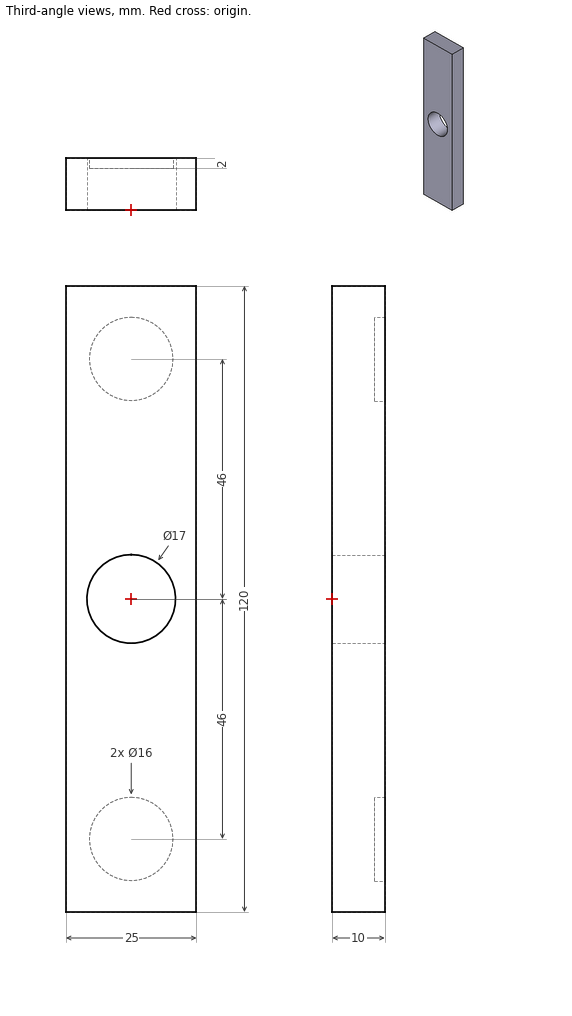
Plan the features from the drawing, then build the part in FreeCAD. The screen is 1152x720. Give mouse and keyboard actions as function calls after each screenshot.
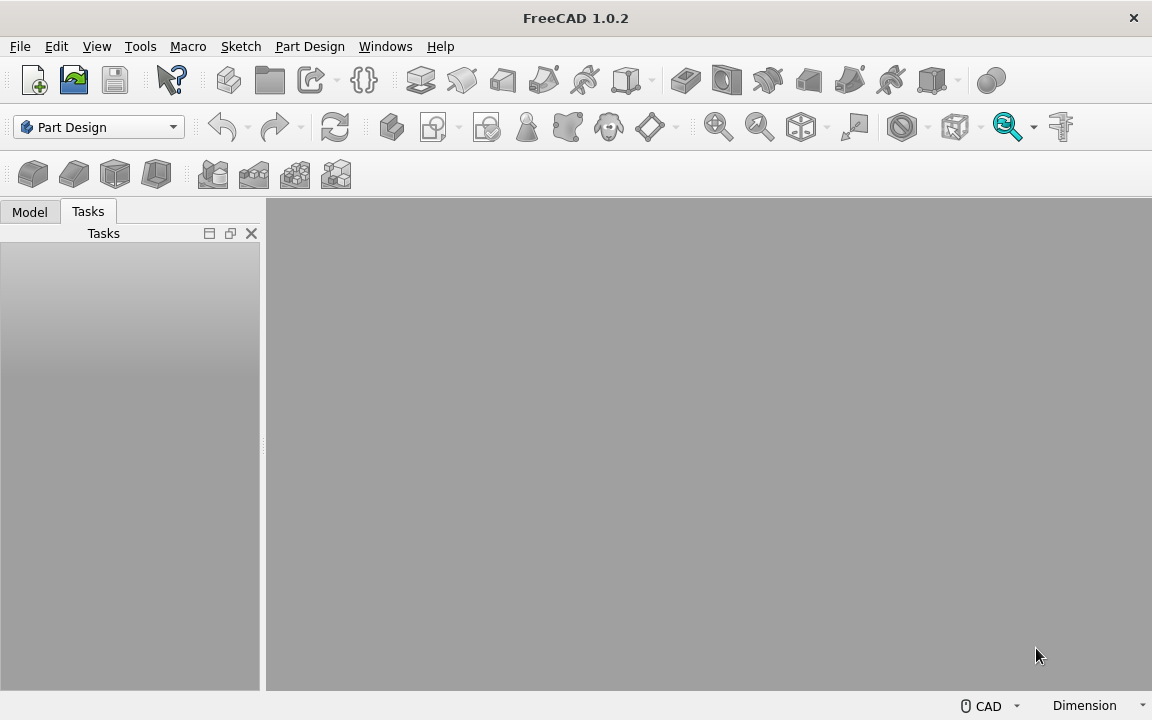
click(33, 80)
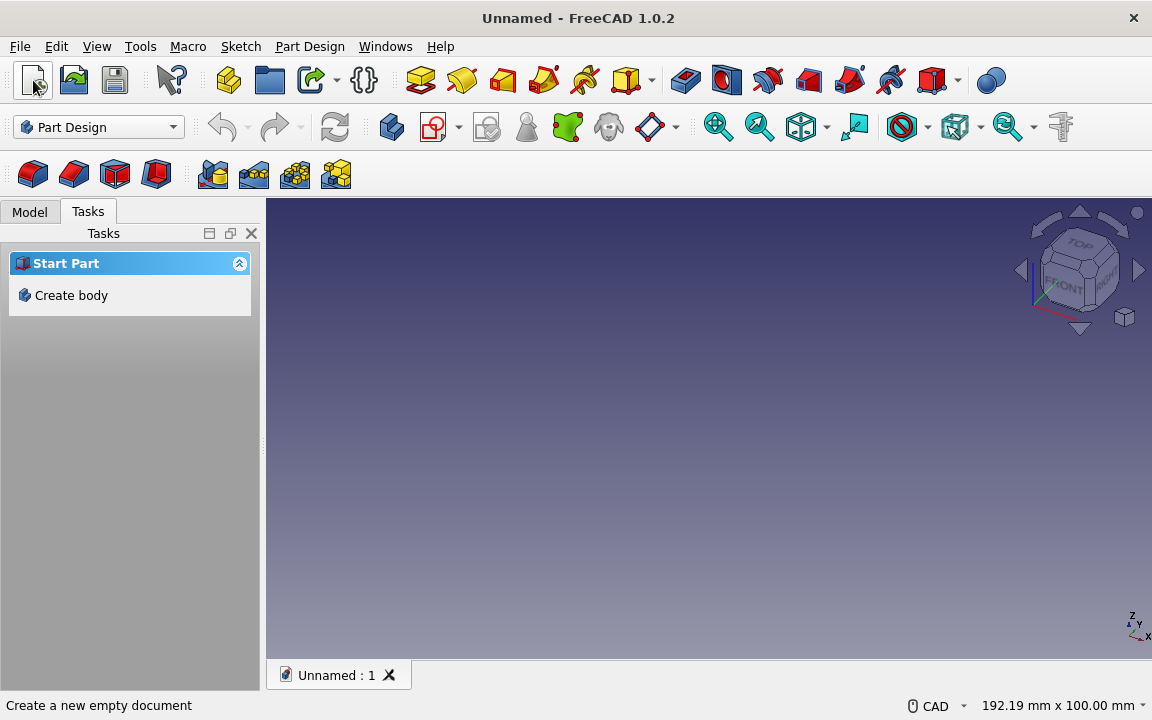
click(432, 128)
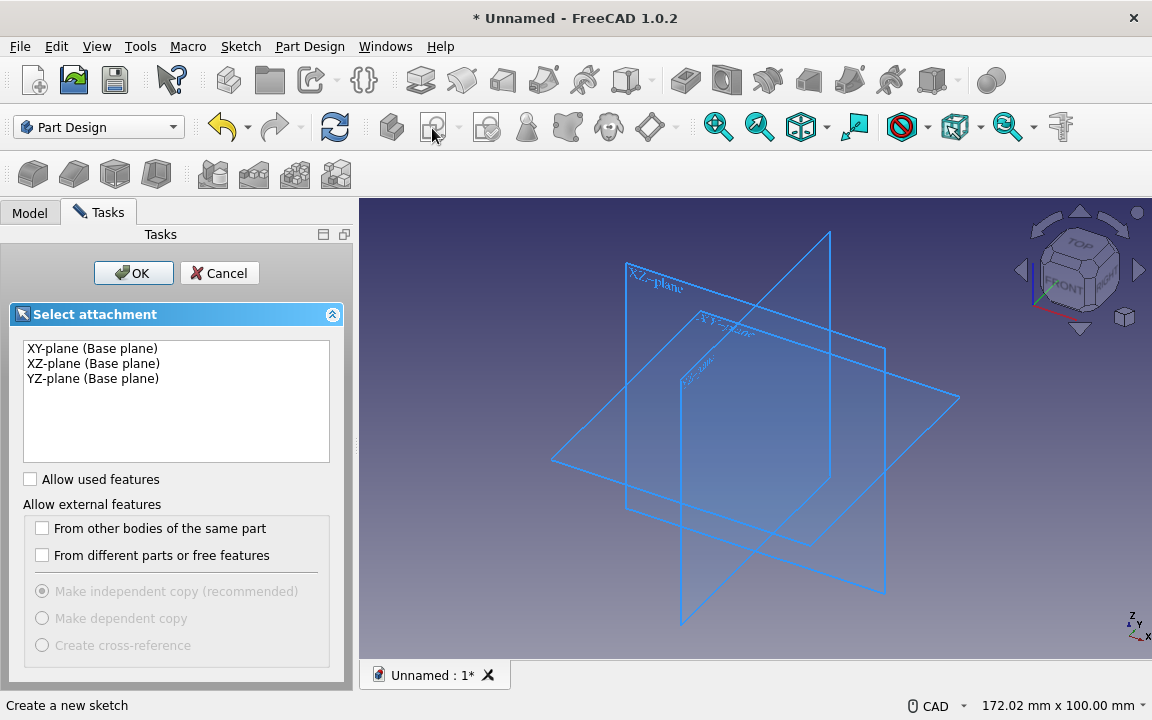
click(84, 364)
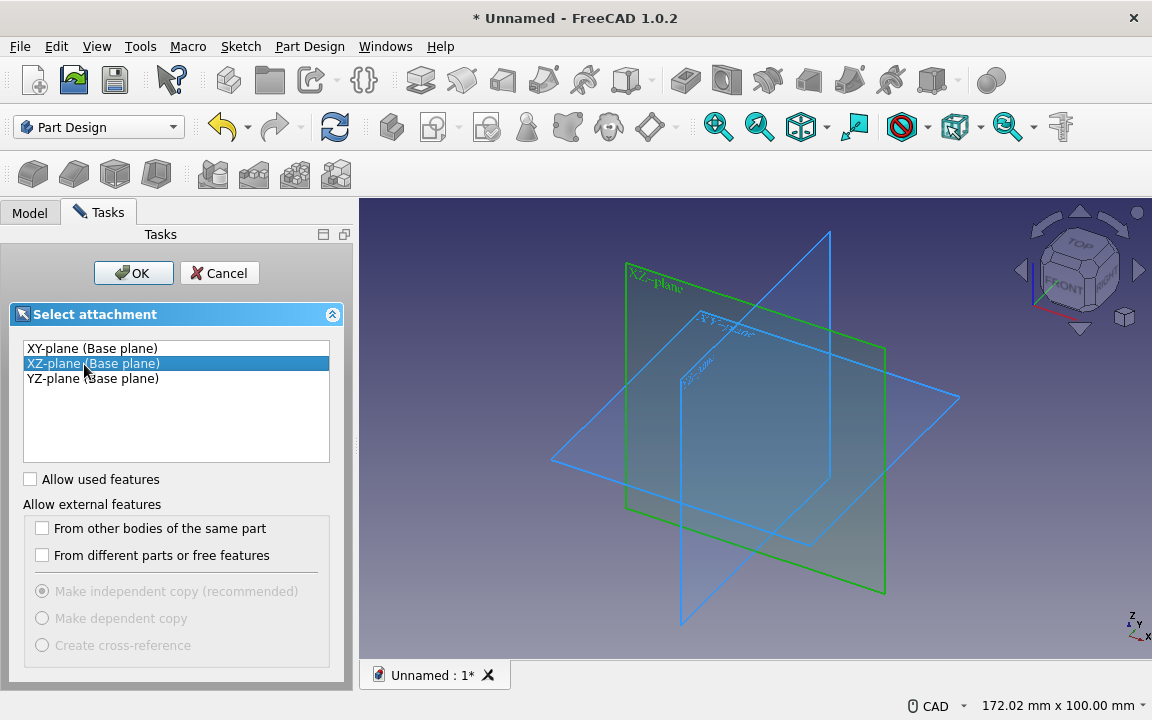
click(134, 273)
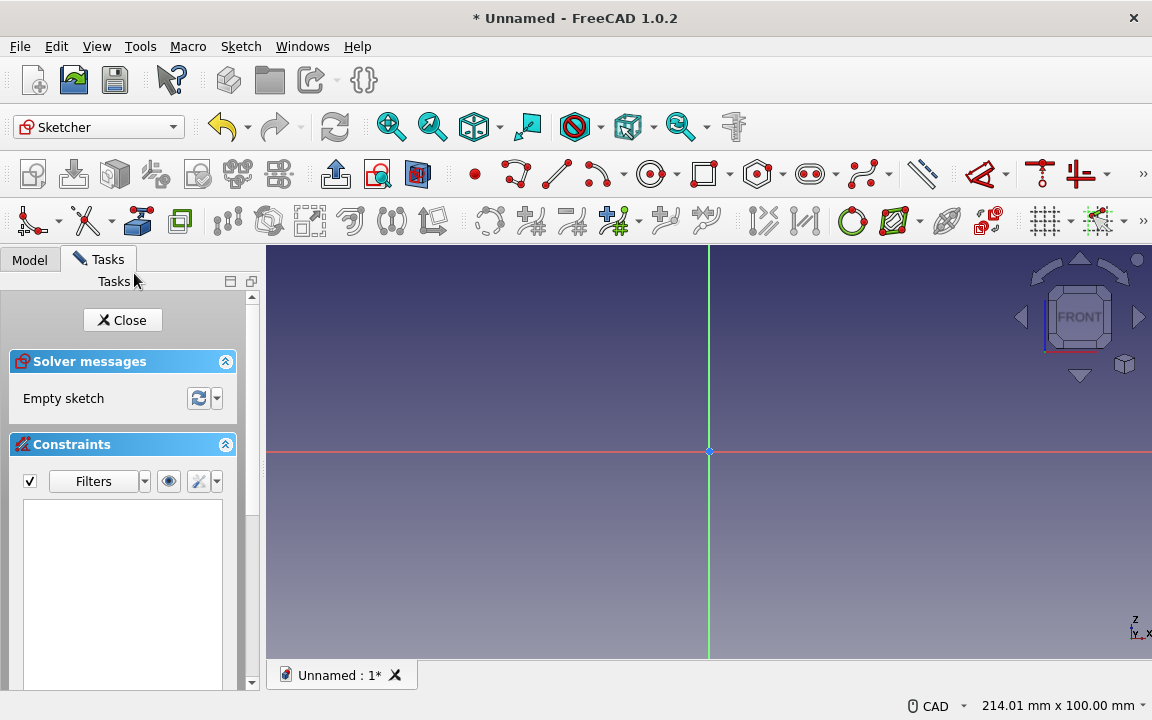
scroll(557, 452, down, 3)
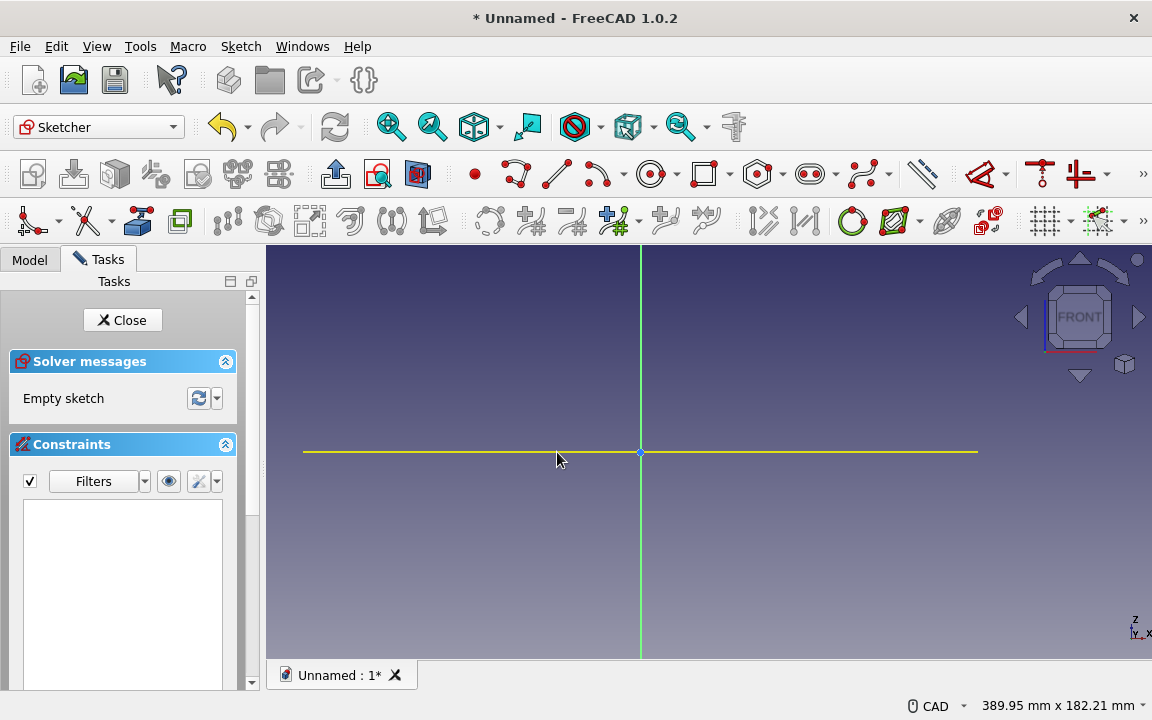
key(g)
key(v)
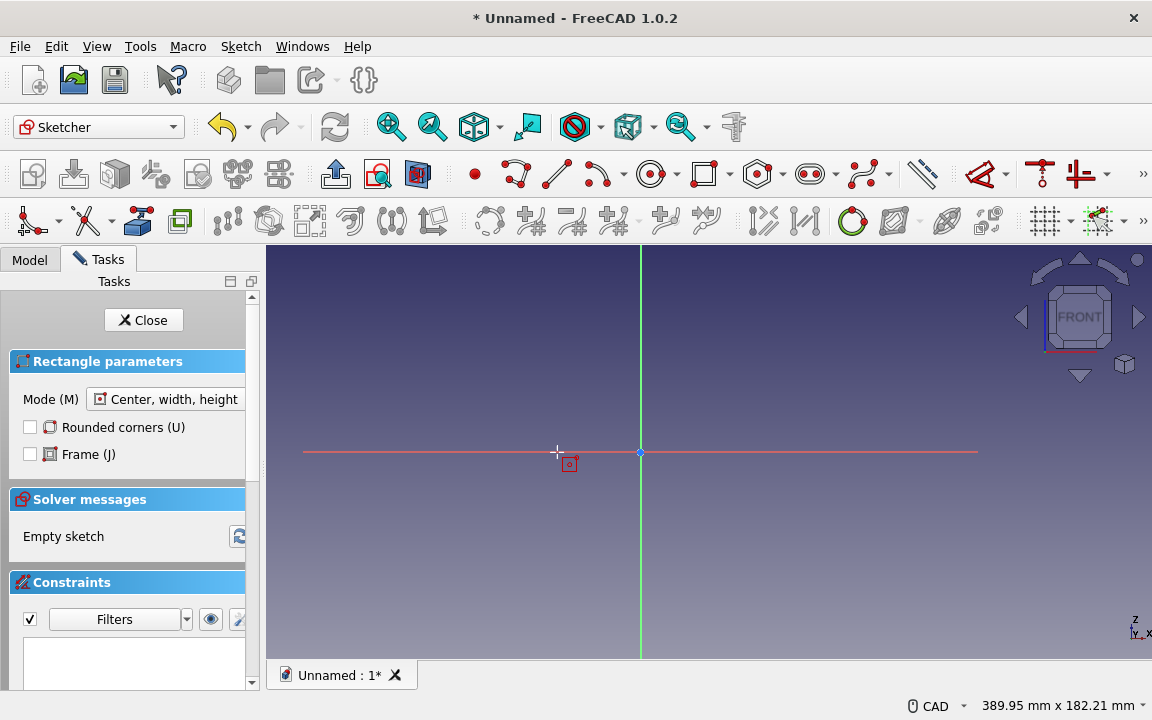
click(641, 452)
move(669, 316)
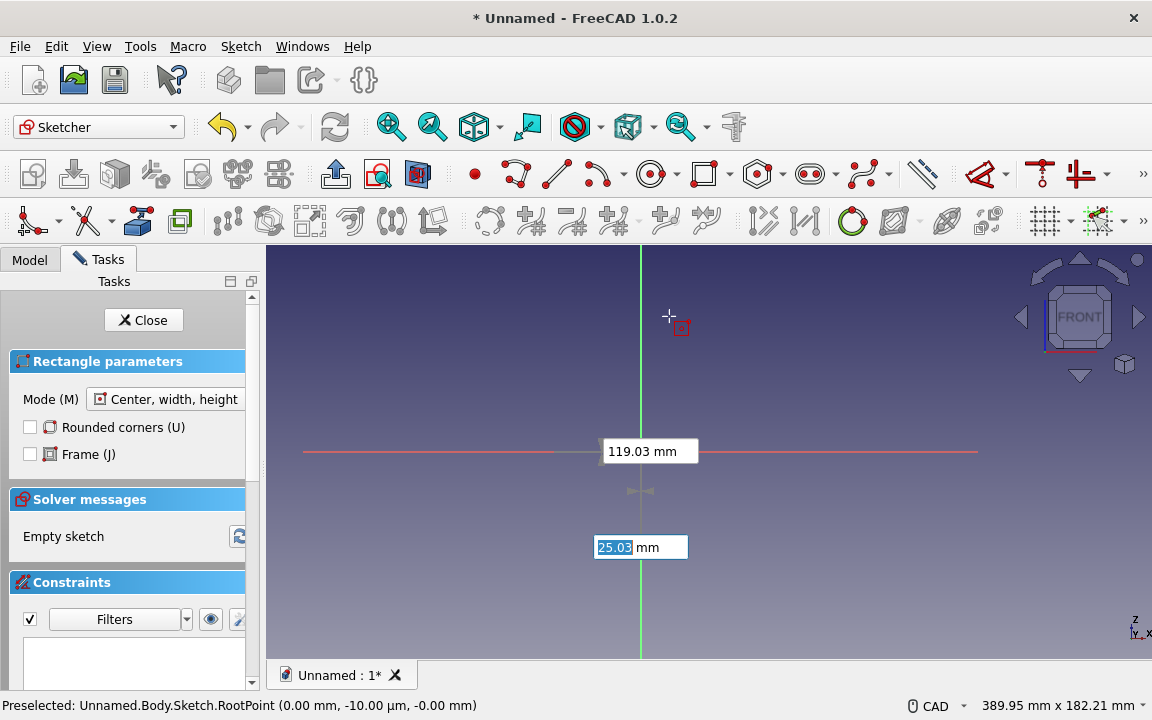
text(25)
key(Tab)
text(120)
key(Return)
key(Escape)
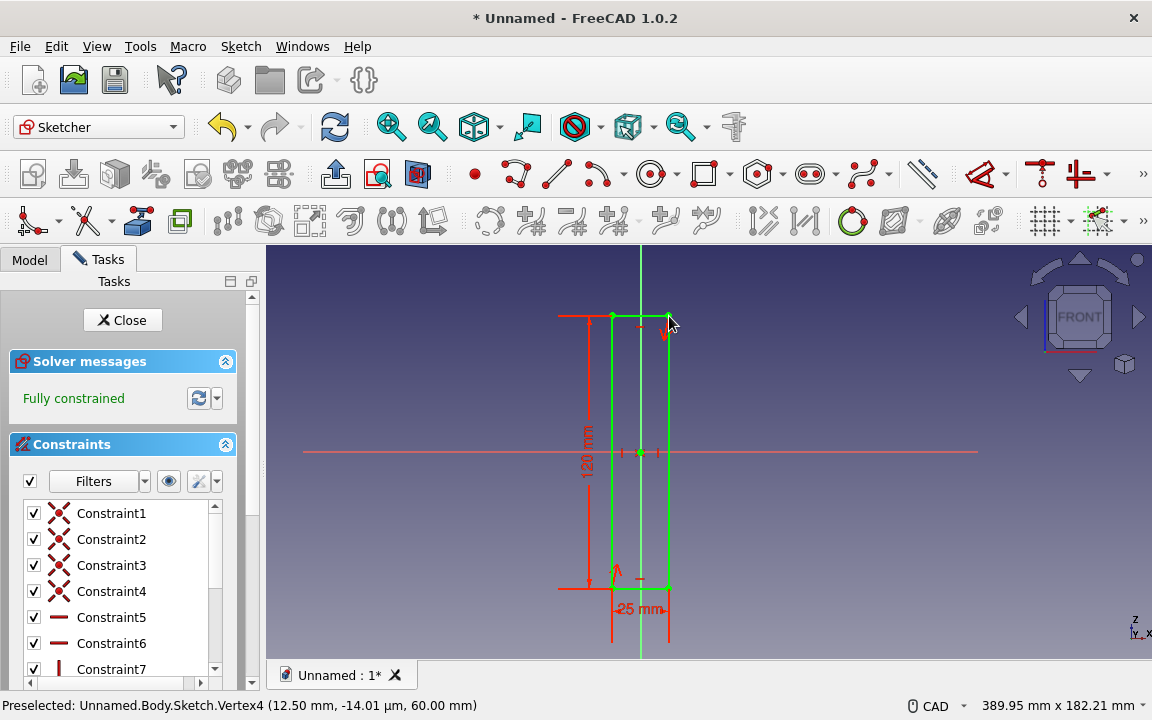
click(123, 320)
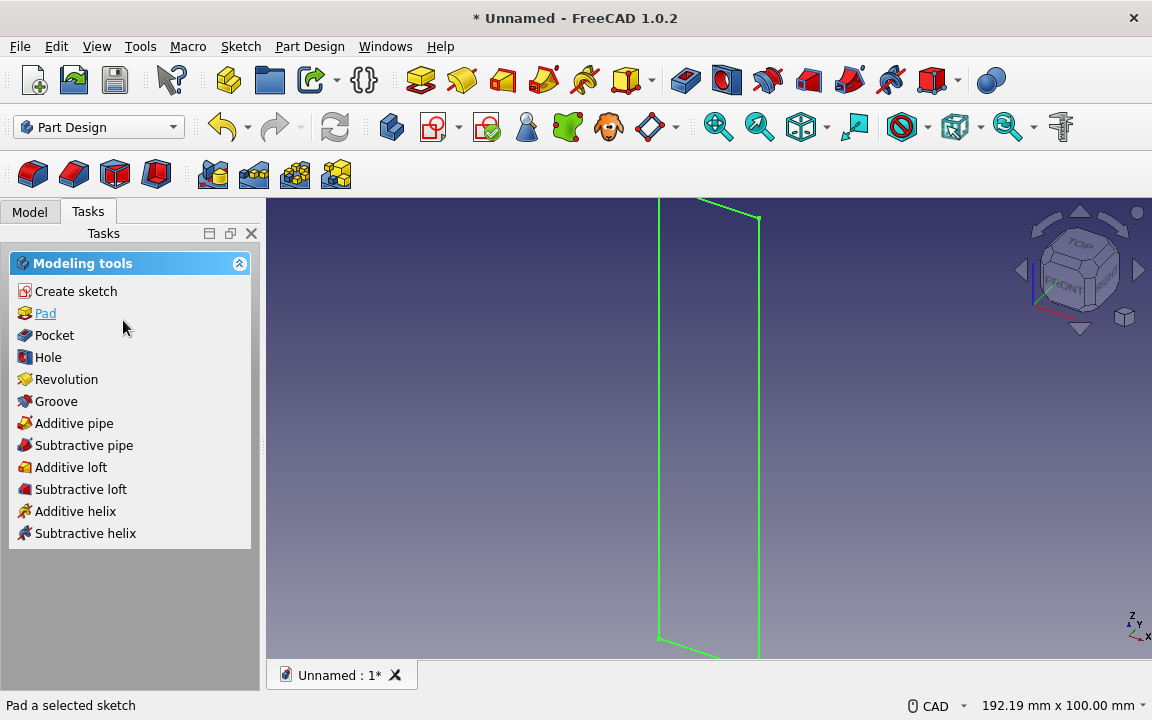
click(421, 80)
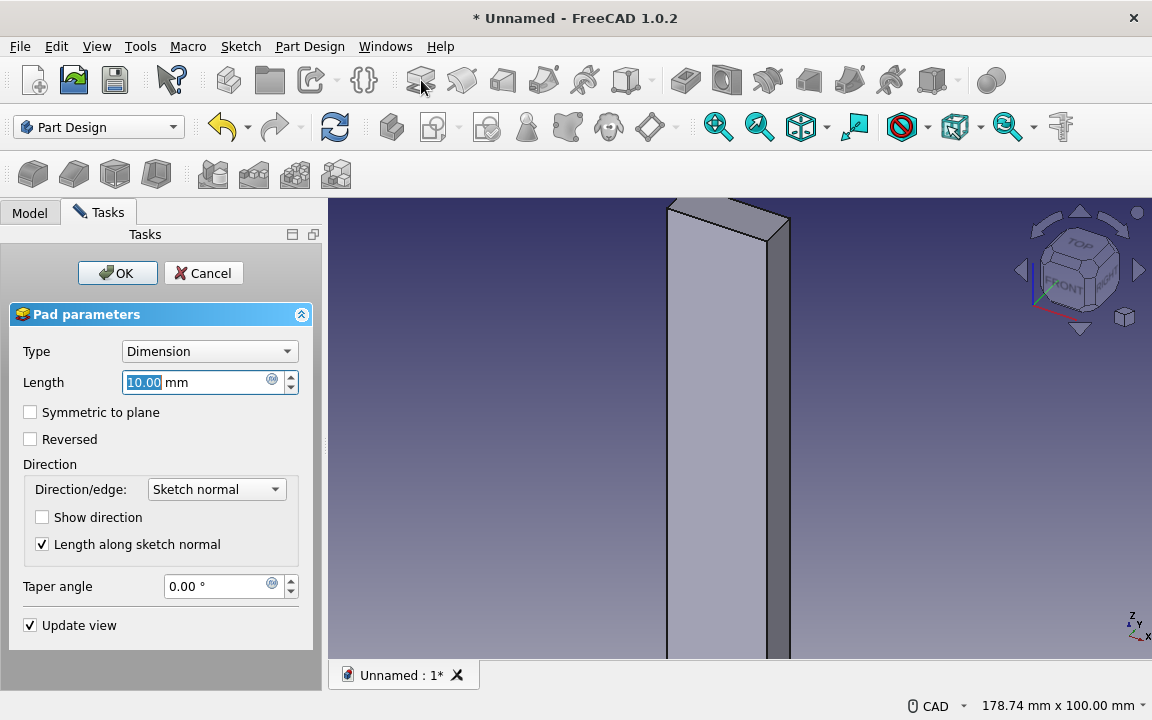
text(10)
key(Tab)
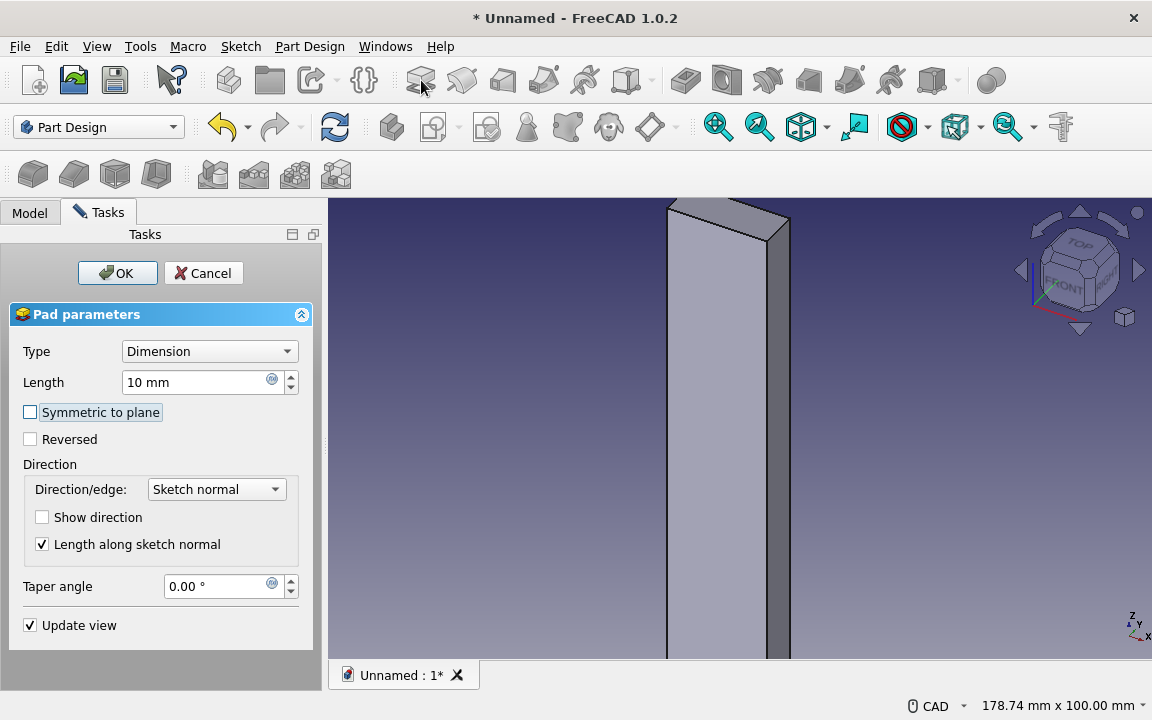
click(31, 439)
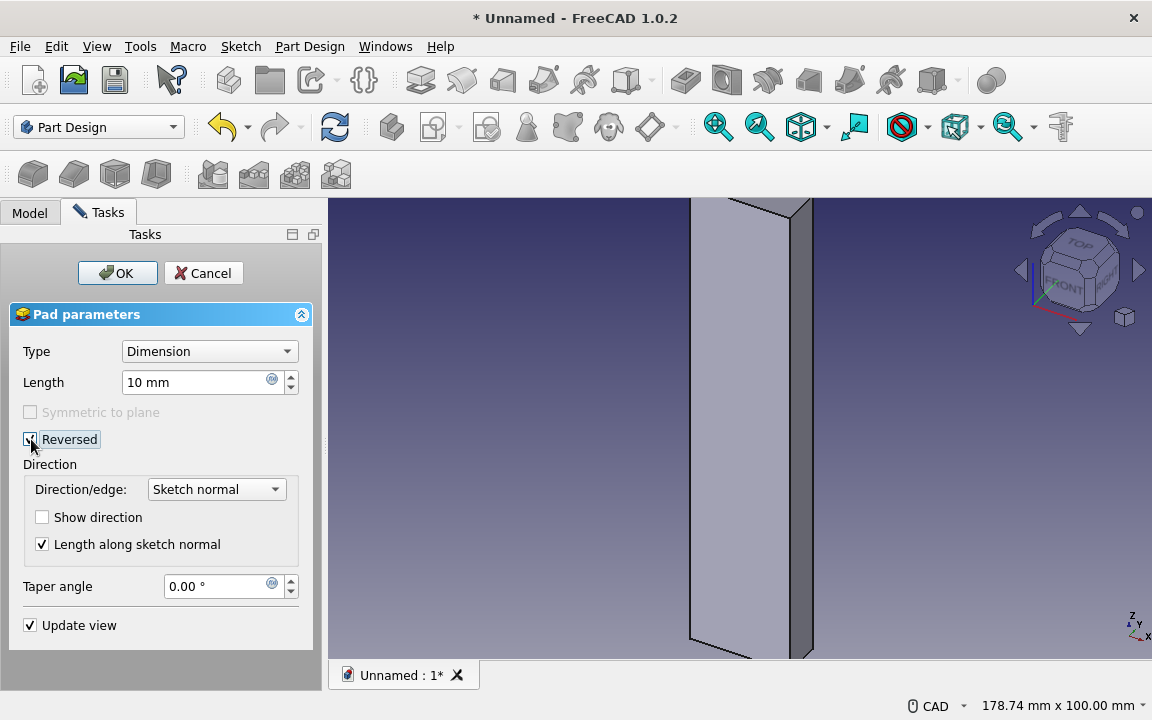
click(118, 273)